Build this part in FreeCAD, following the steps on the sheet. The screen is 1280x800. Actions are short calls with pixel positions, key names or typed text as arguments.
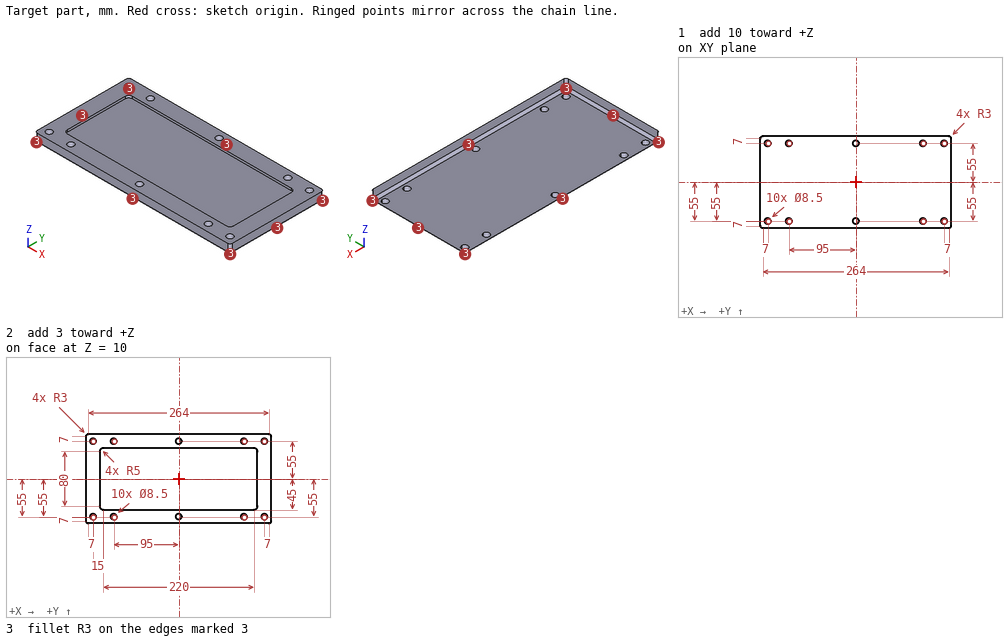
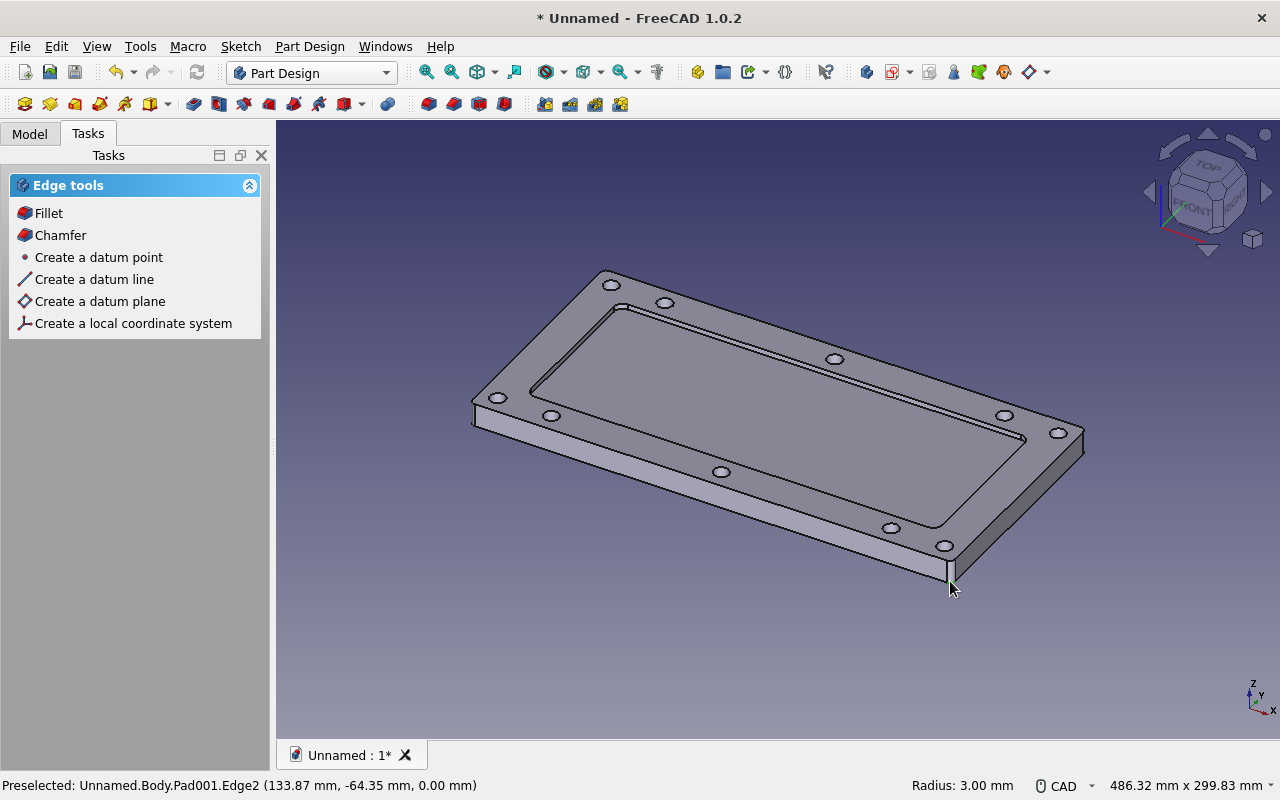
key(0)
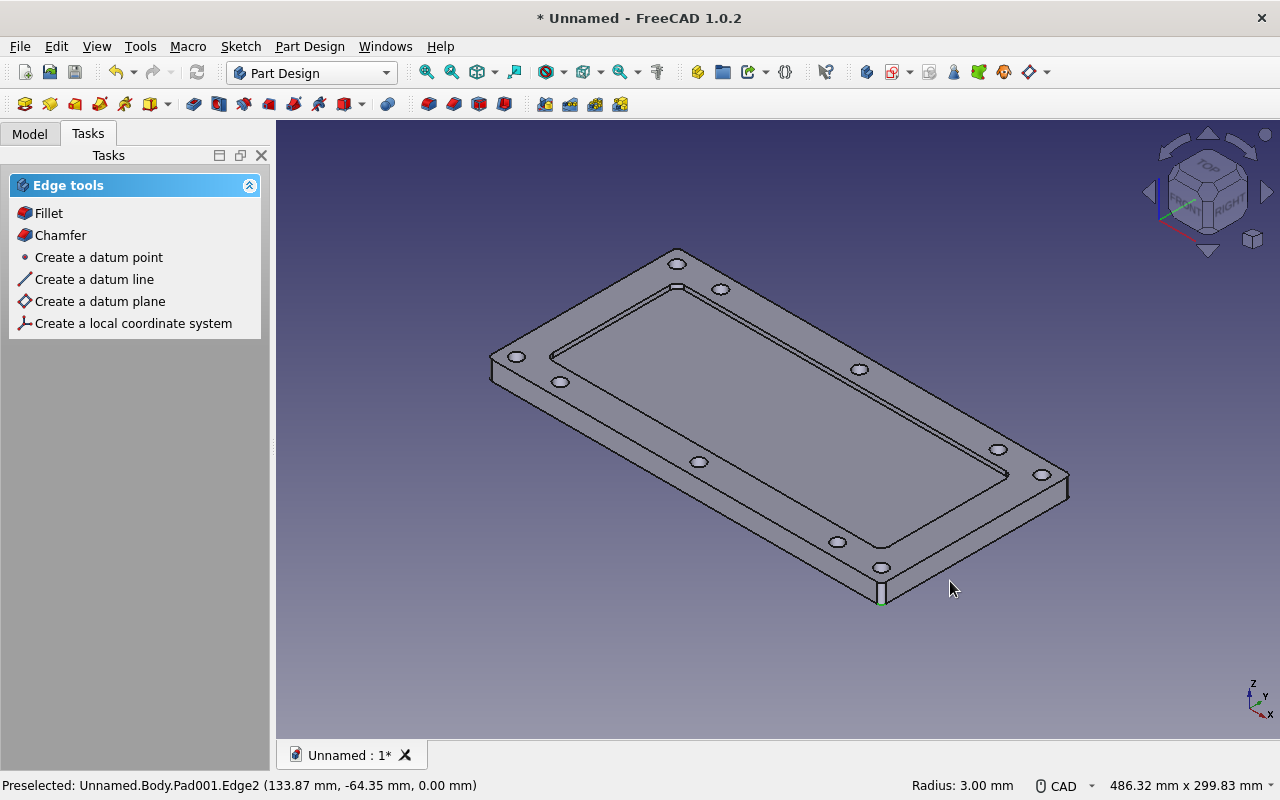
key(2)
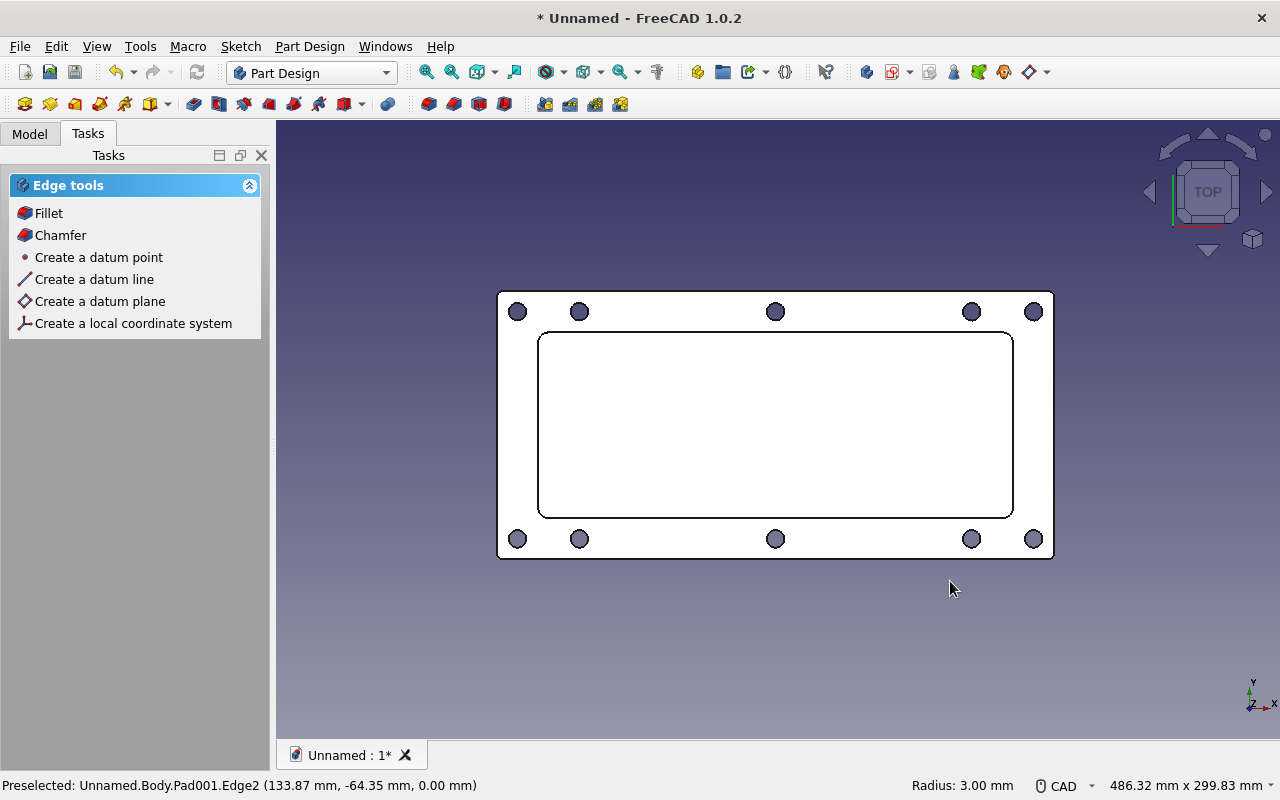
key(1)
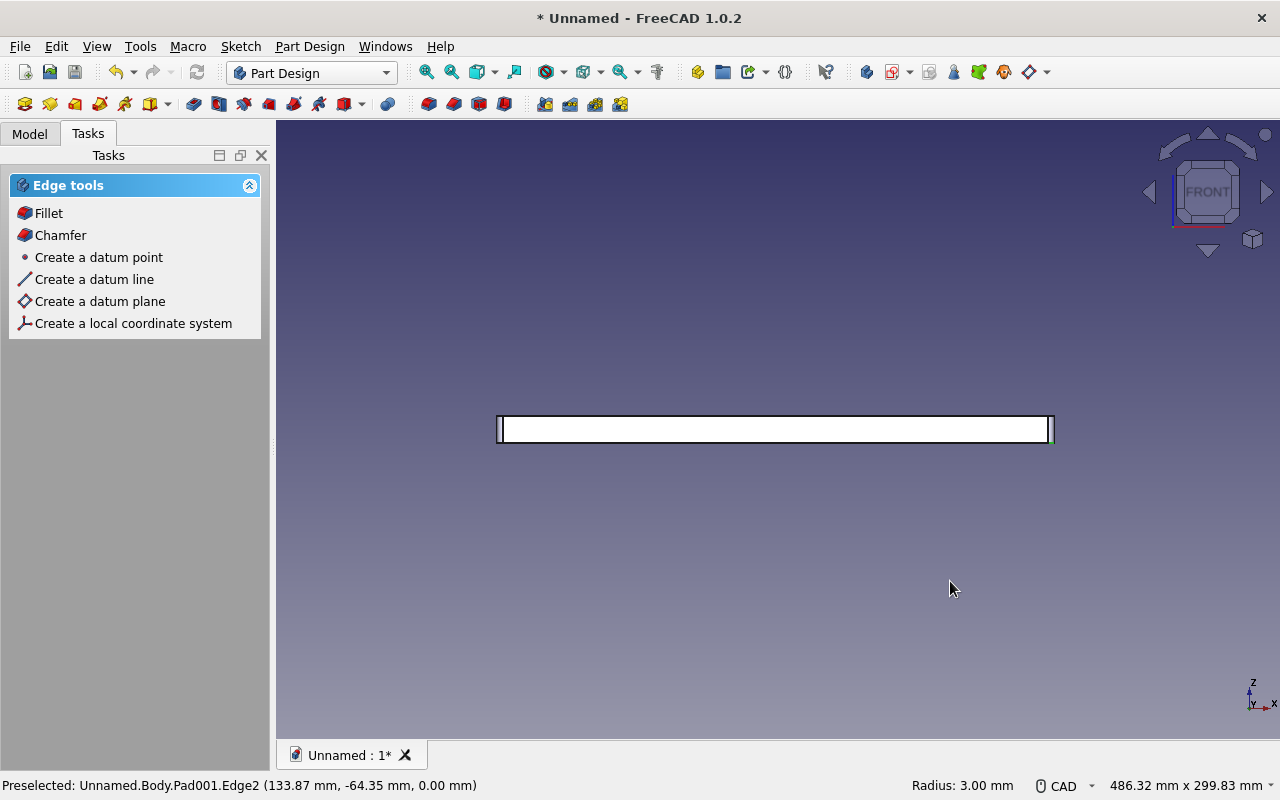
click(776, 442, ctrl)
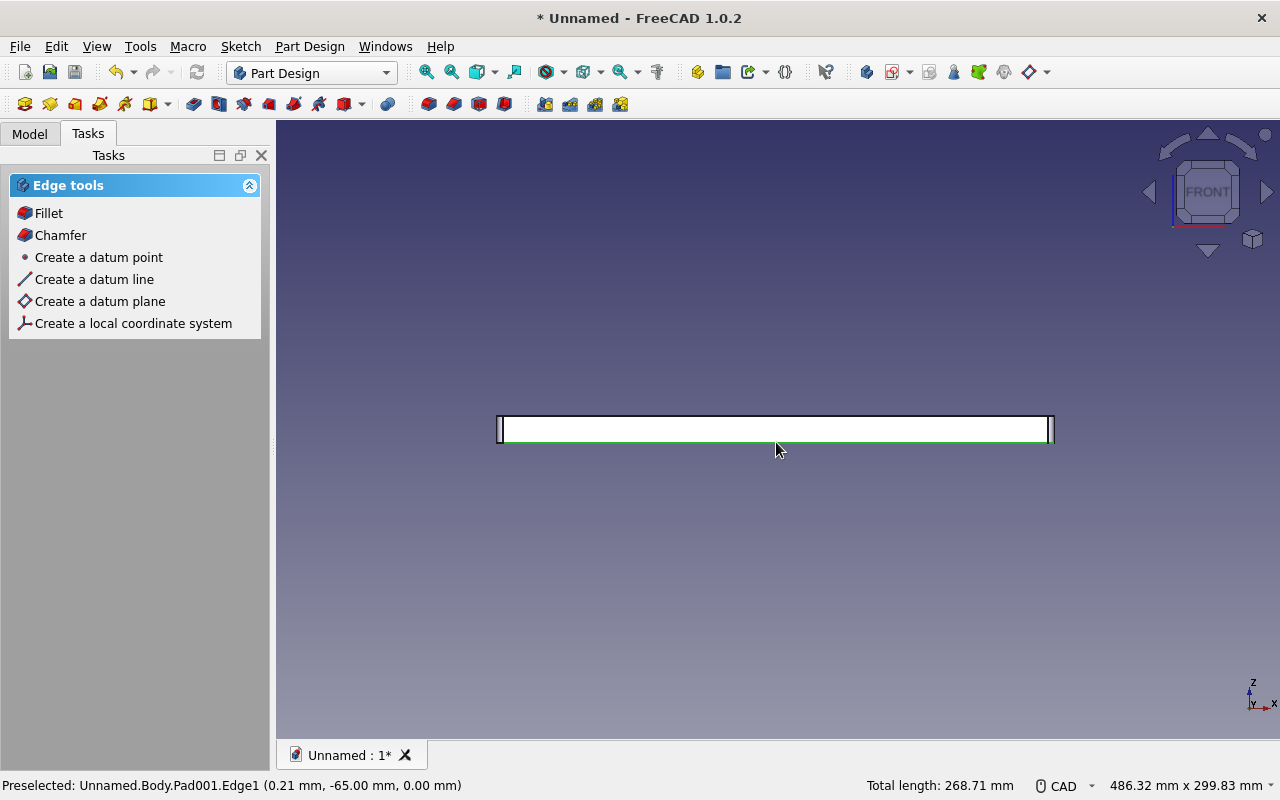
click(497, 442, ctrl)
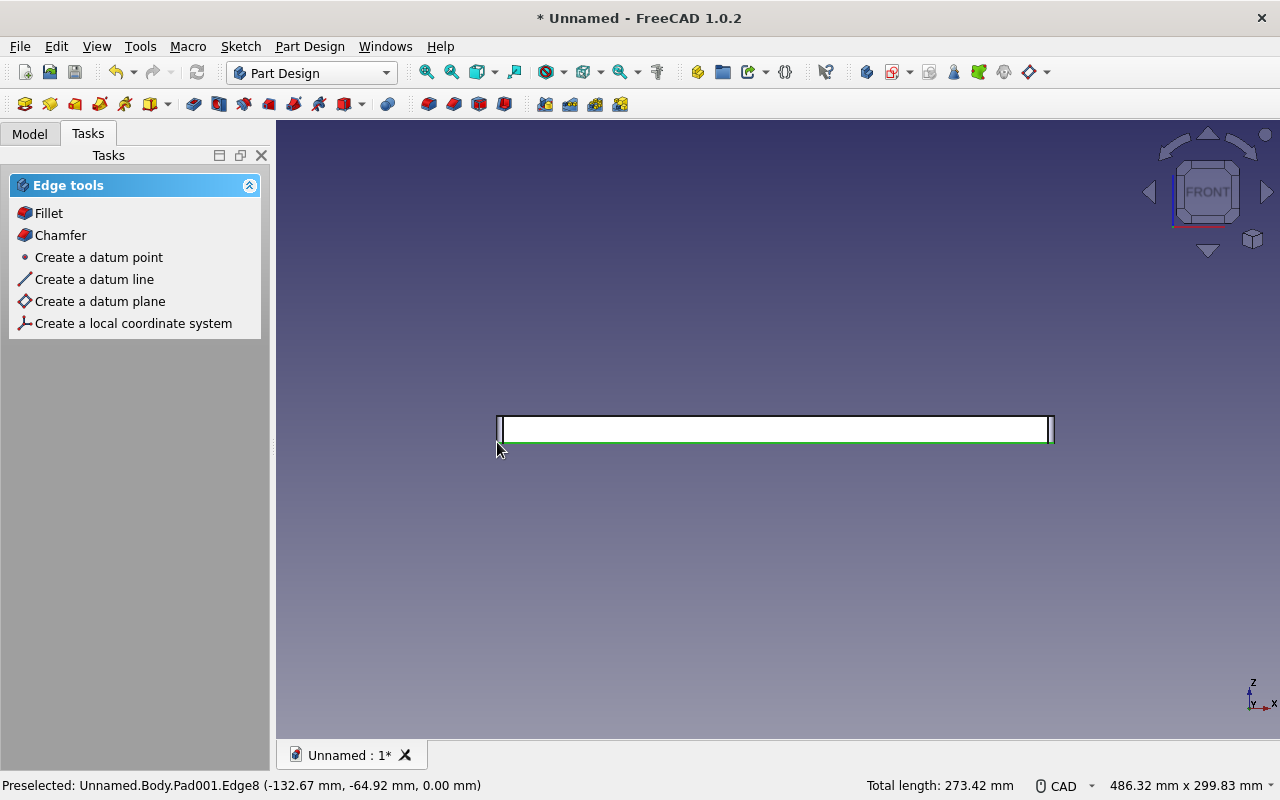
key(3)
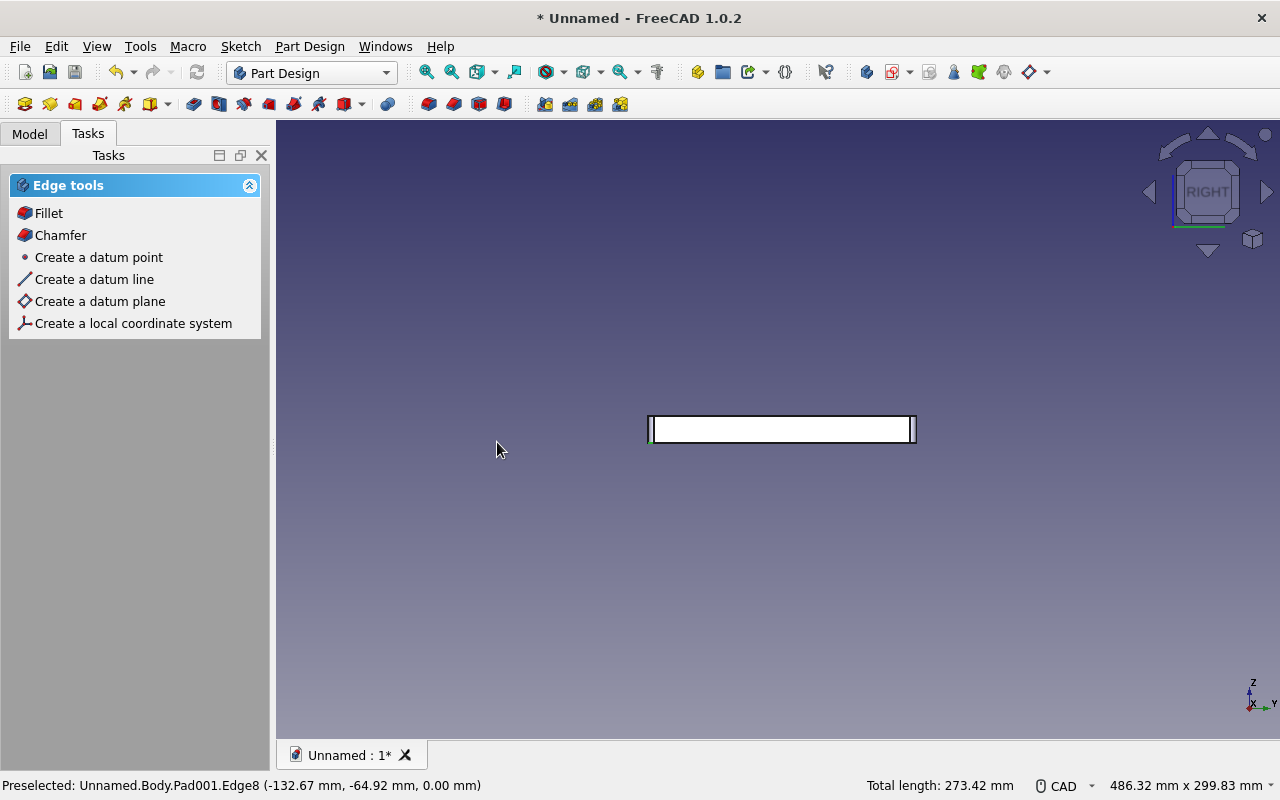
click(427, 72)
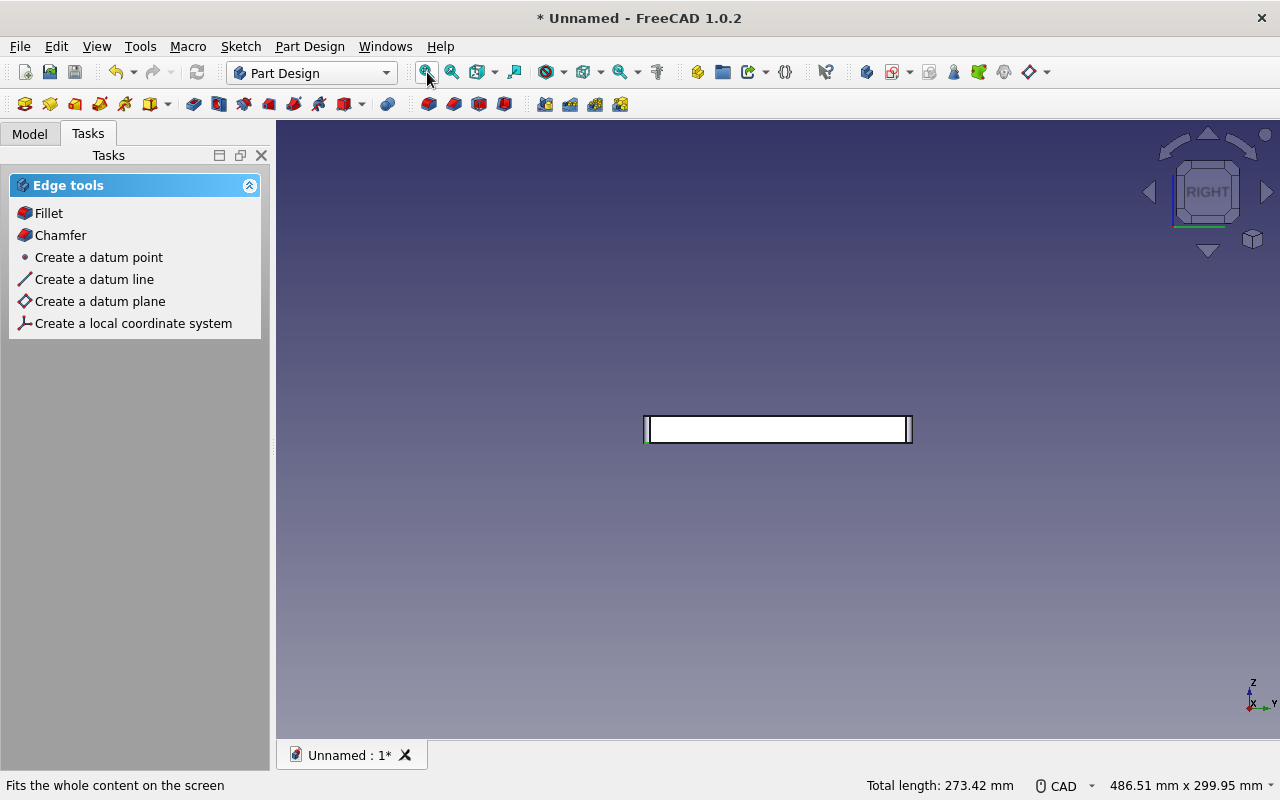
click(912, 442, ctrl)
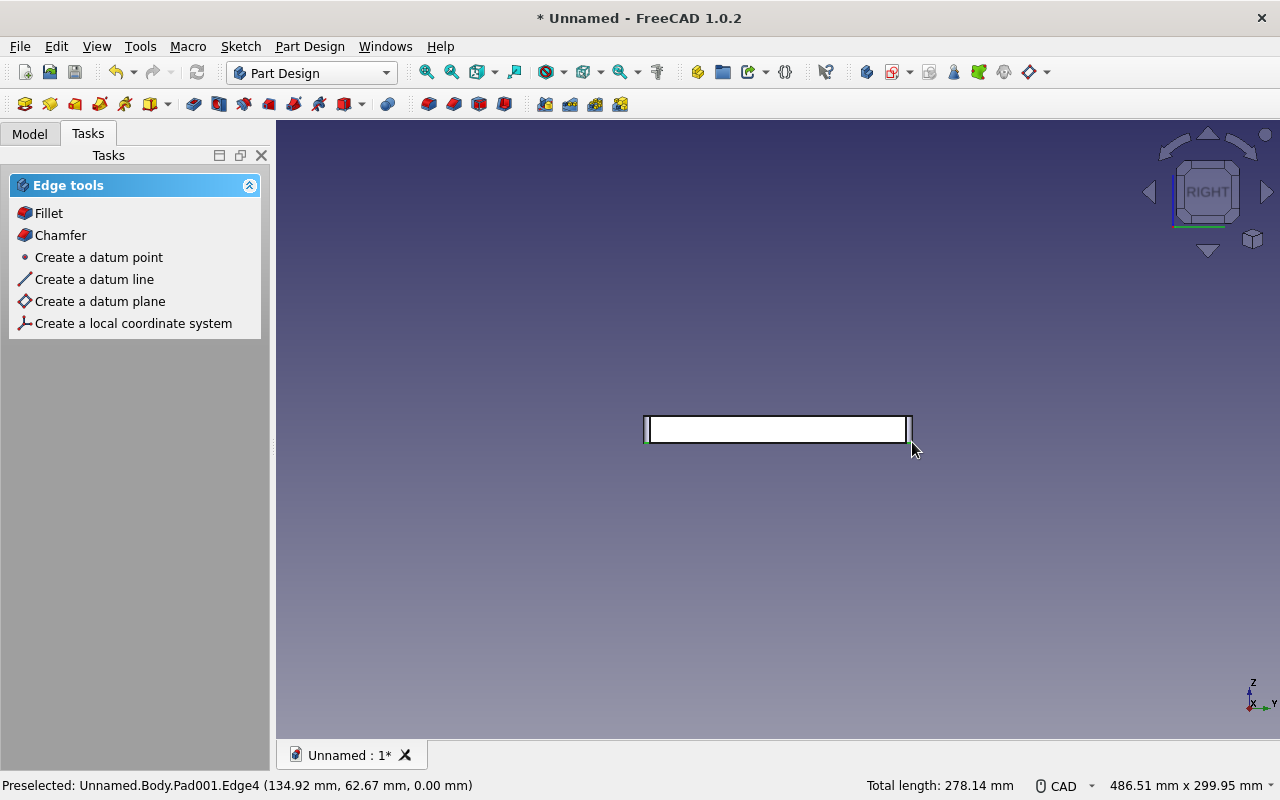
click(778, 442, ctrl)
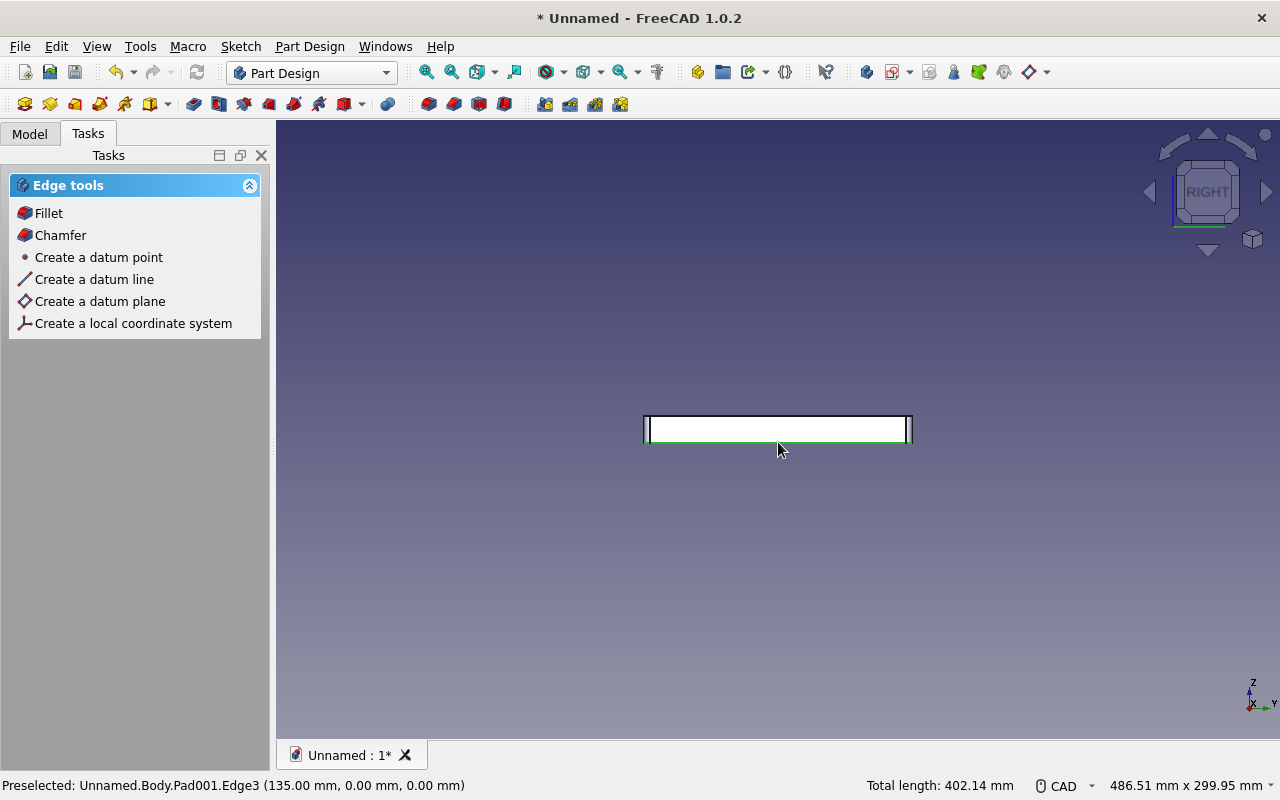
key(5)